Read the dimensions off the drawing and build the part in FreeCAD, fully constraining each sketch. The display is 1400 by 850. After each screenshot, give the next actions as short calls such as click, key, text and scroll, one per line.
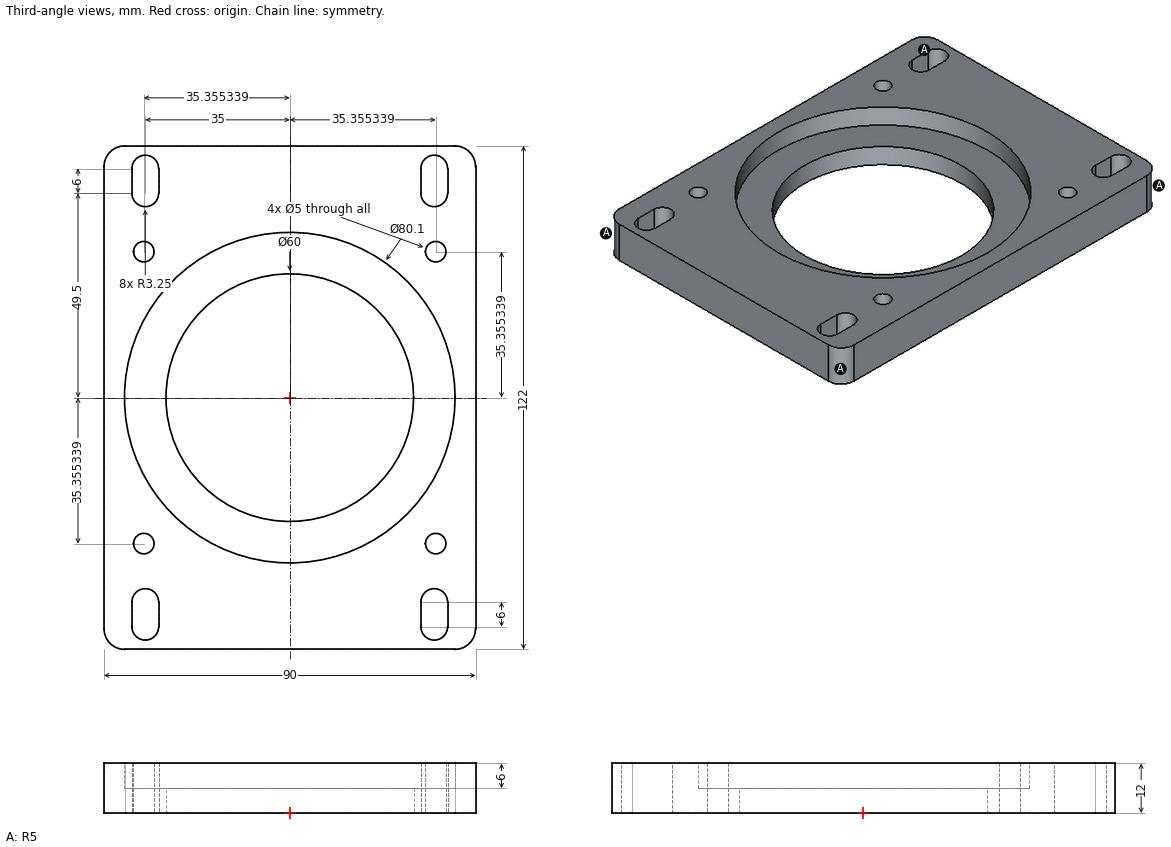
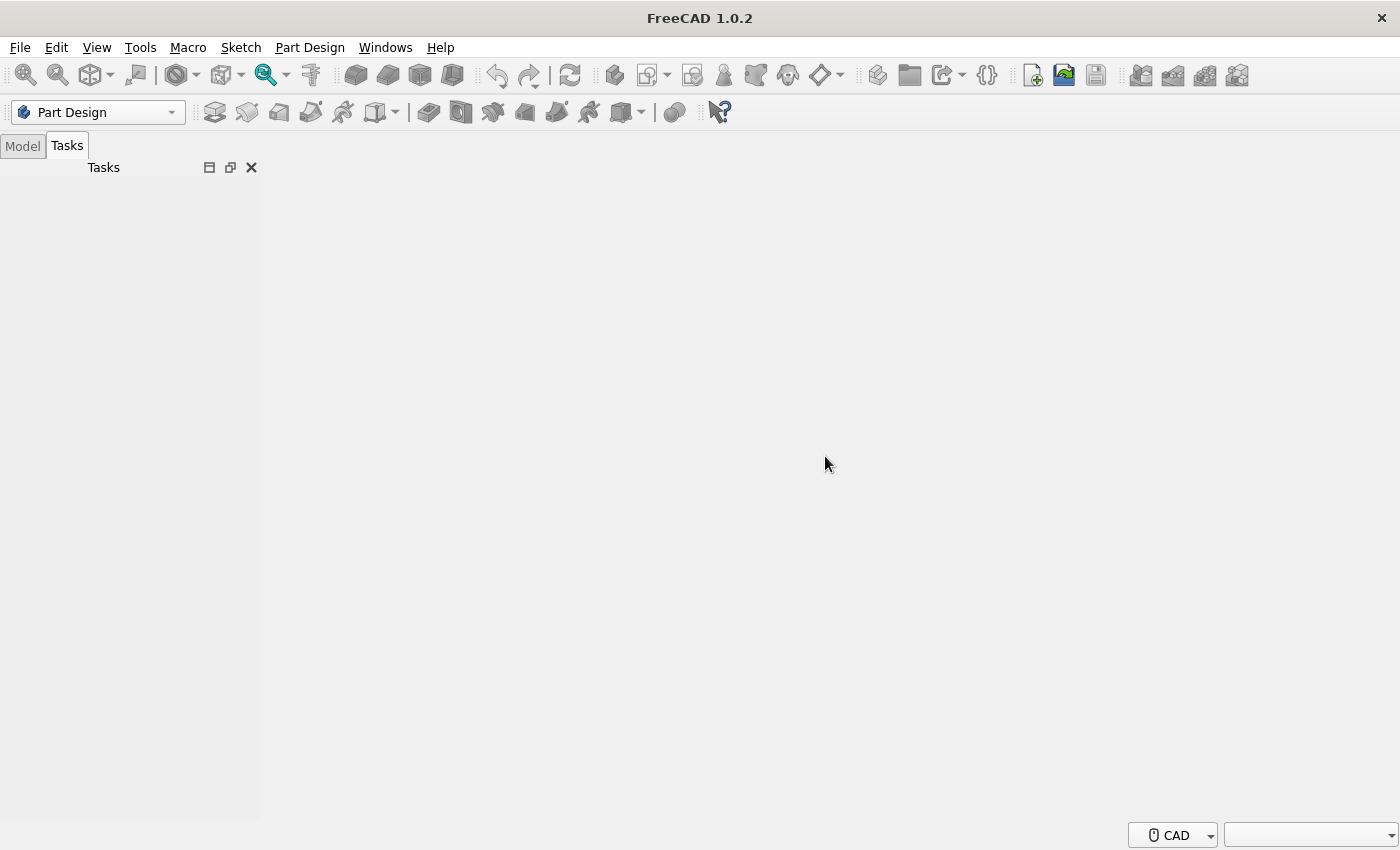
click(1032, 76)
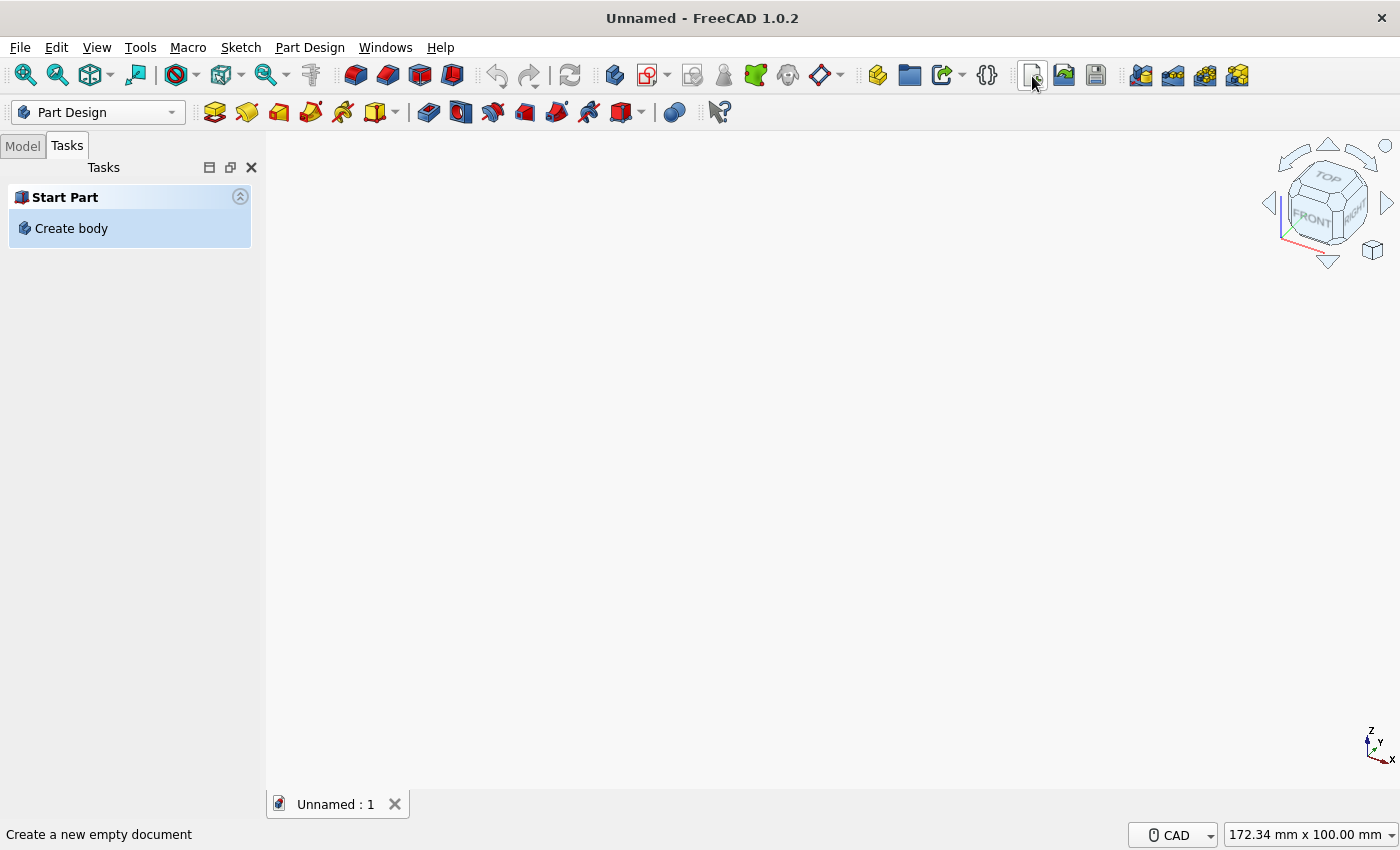
click(648, 76)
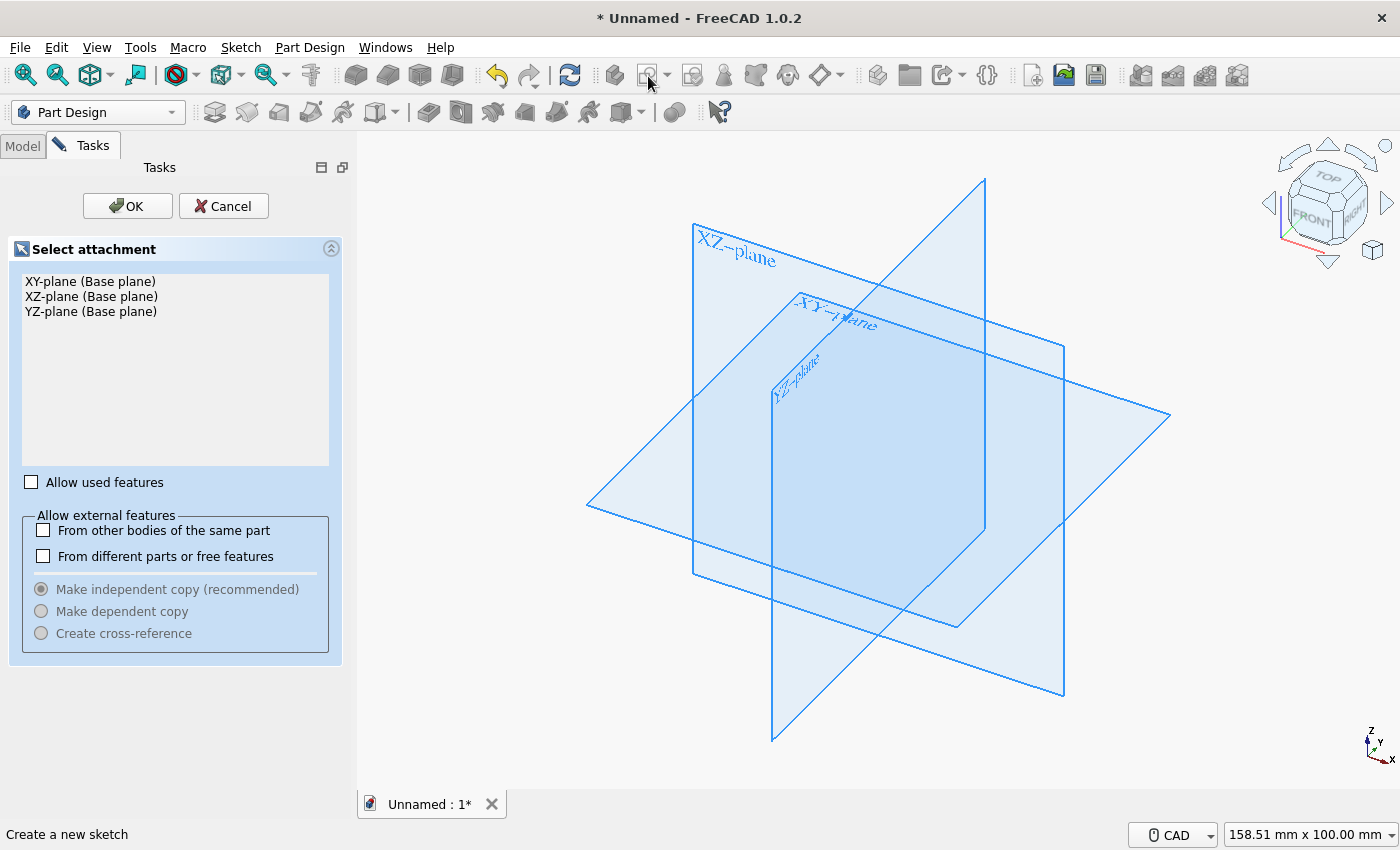
click(82, 282)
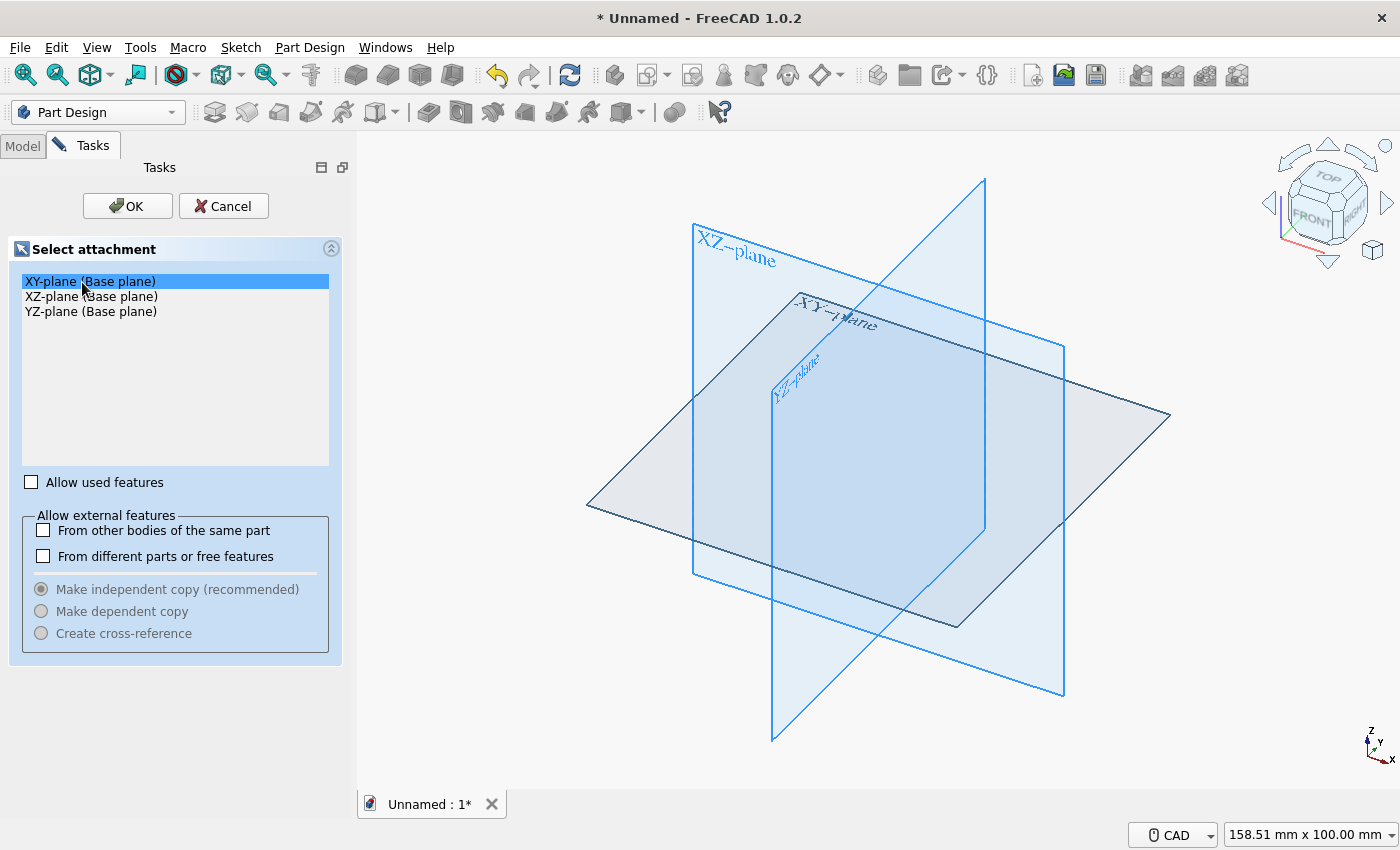
click(128, 206)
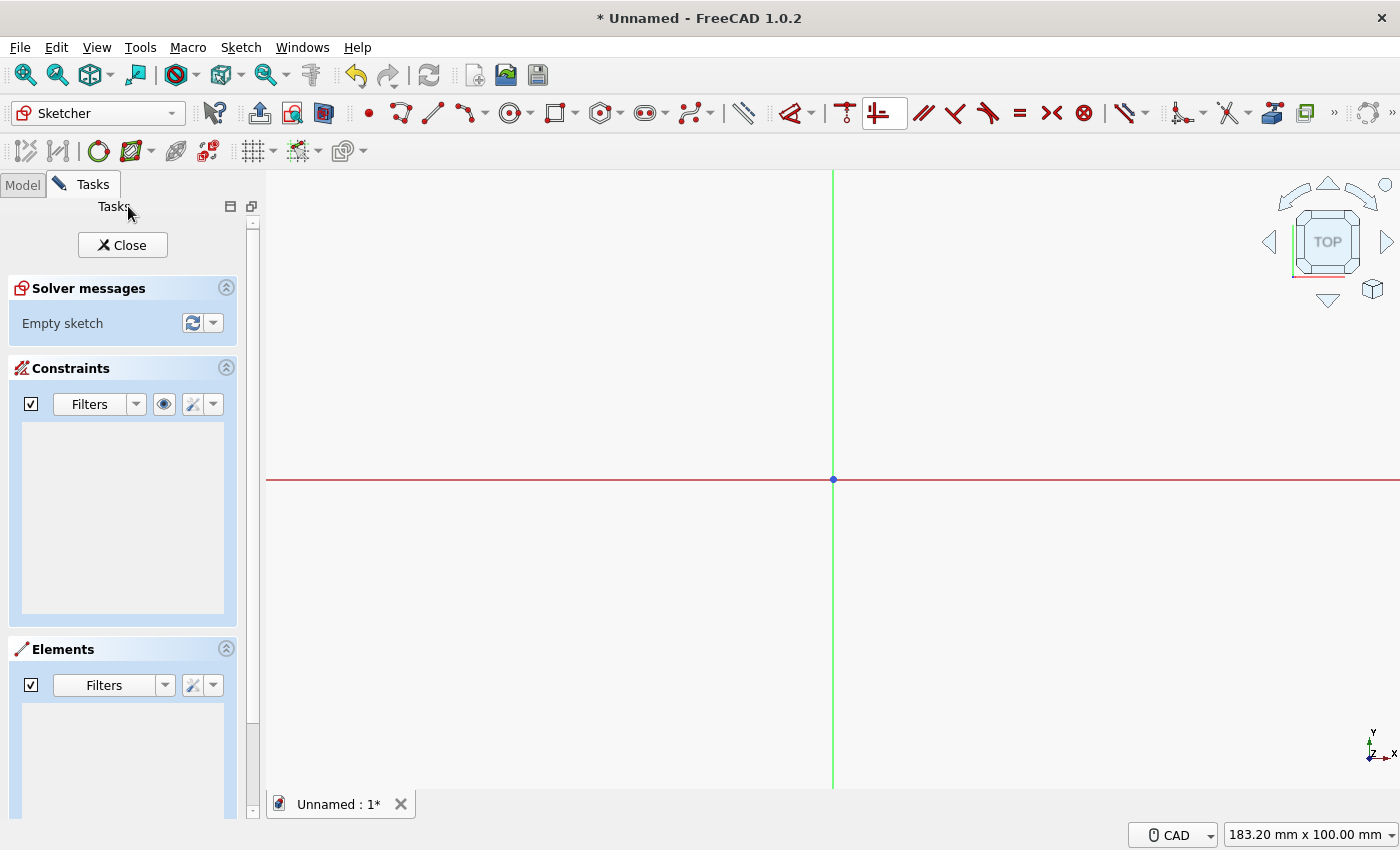
scroll(681, 479, down, 3)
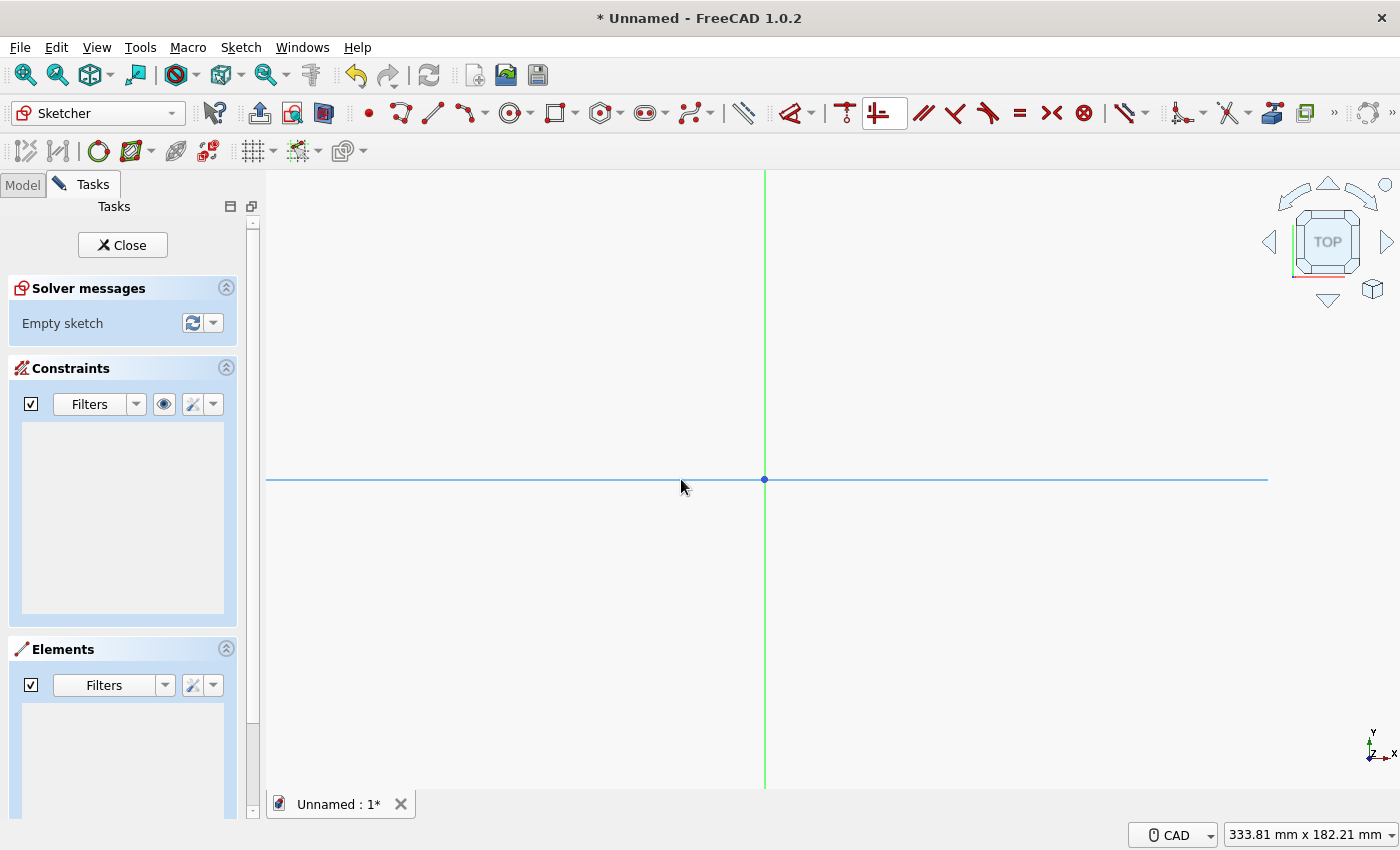
key(g)
key(v)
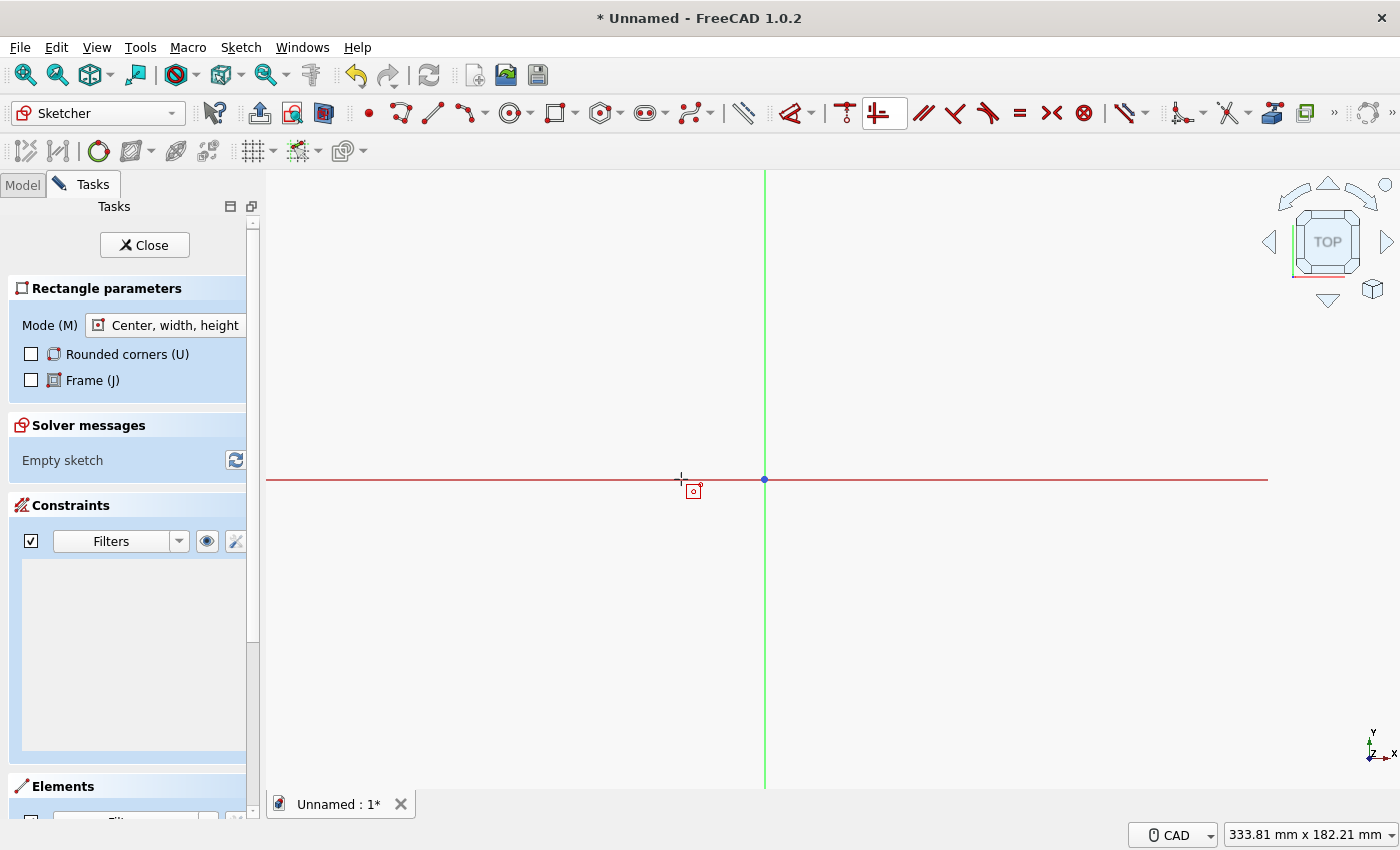
click(765, 480)
move(917, 272)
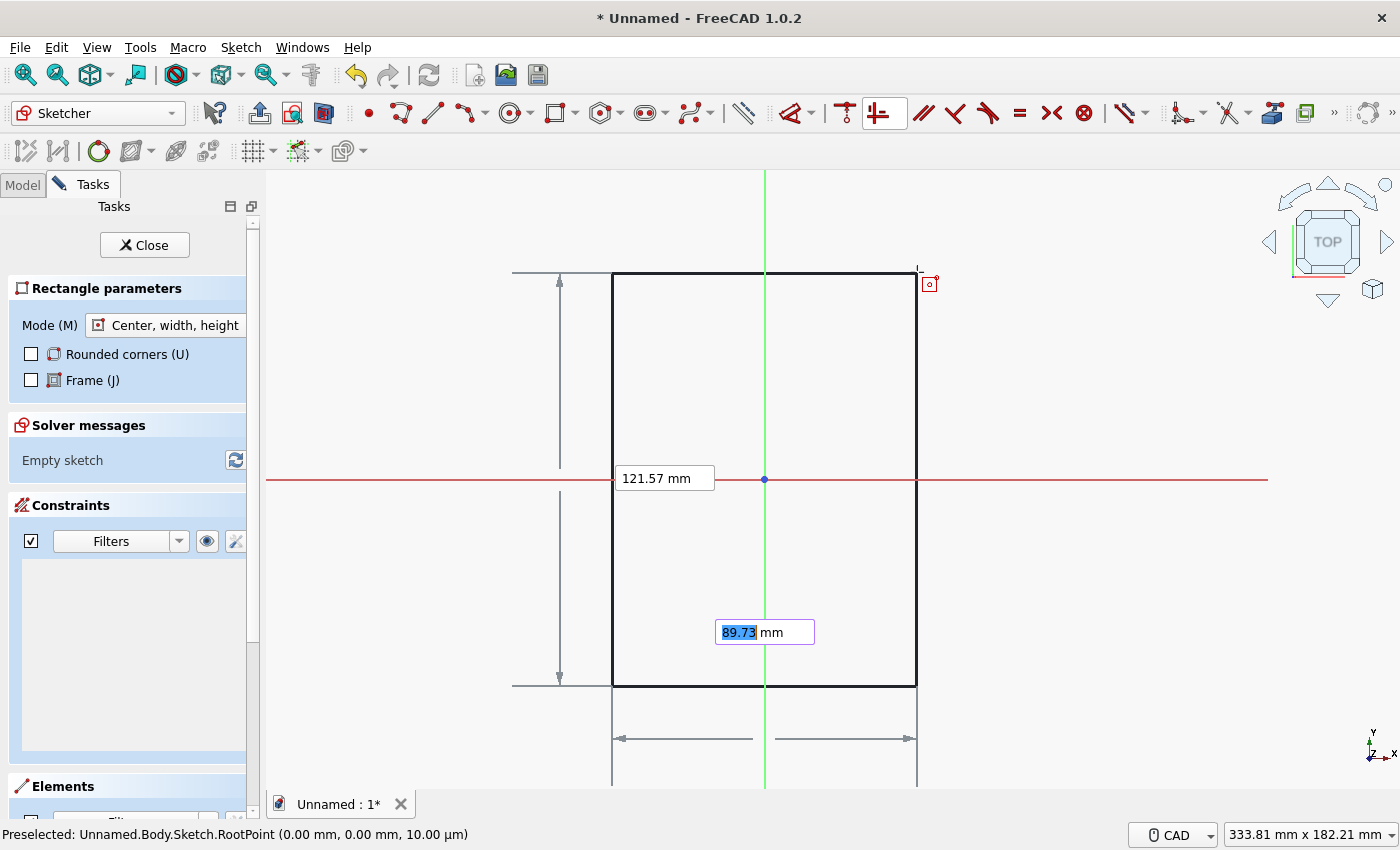
text(90)
key(Tab)
text(122)
key(Return)
key(Escape)